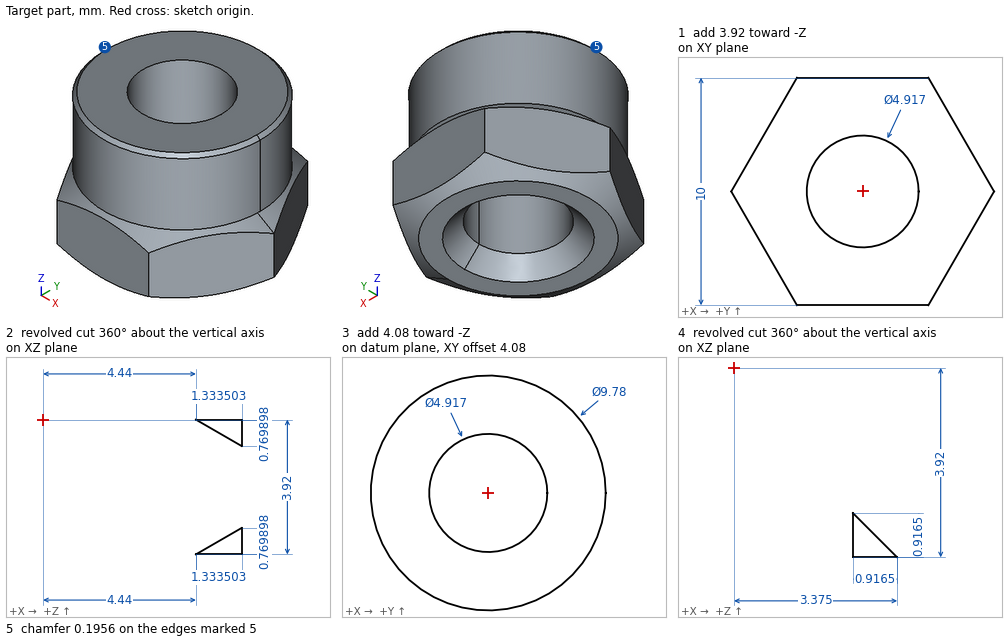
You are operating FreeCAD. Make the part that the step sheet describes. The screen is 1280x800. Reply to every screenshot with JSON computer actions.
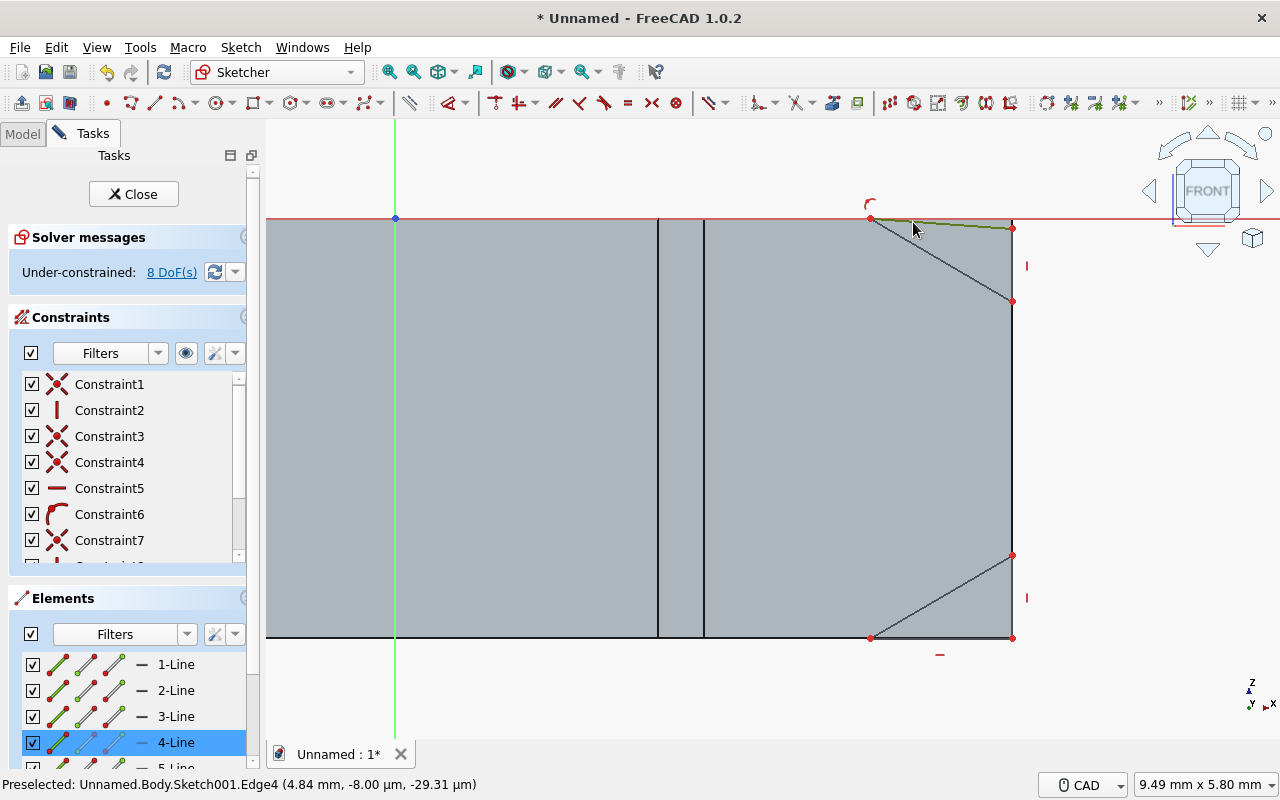
{"action": "key", "text": "h"}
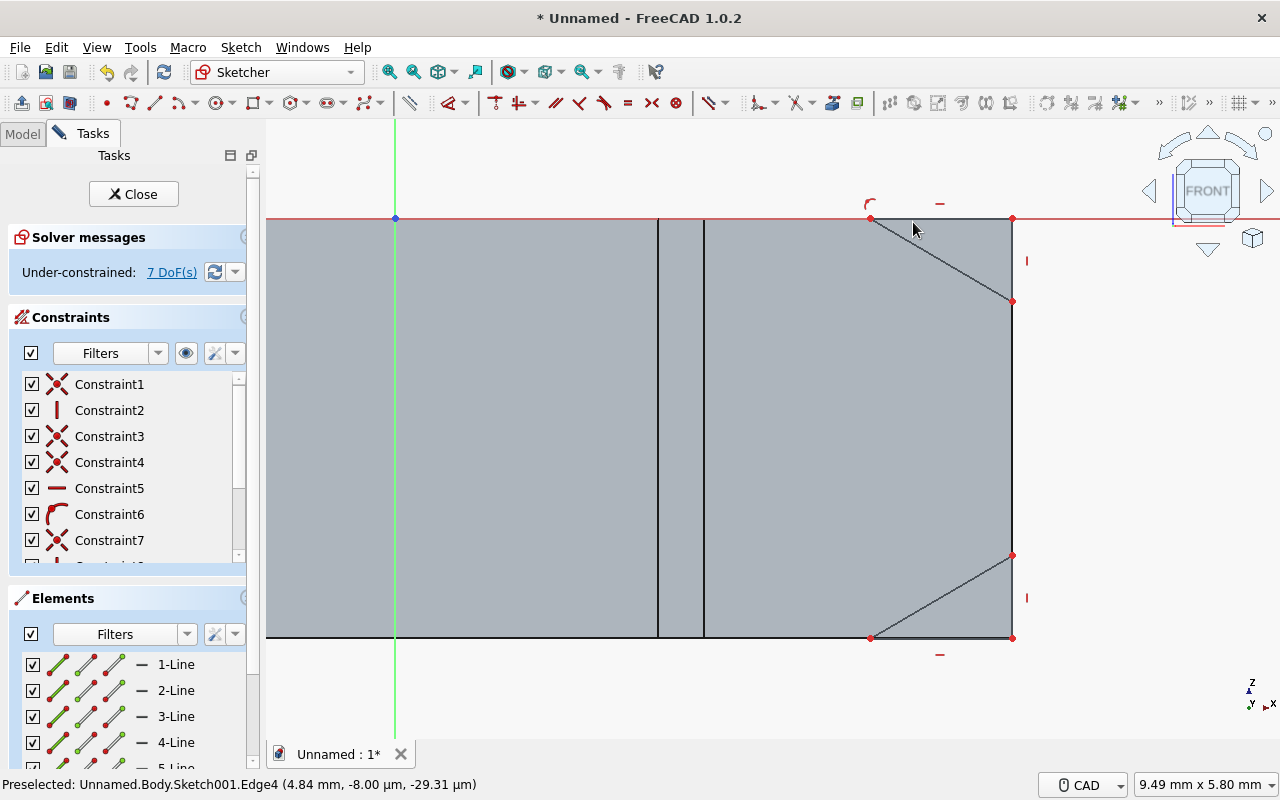
{"action": "key", "text": "d"}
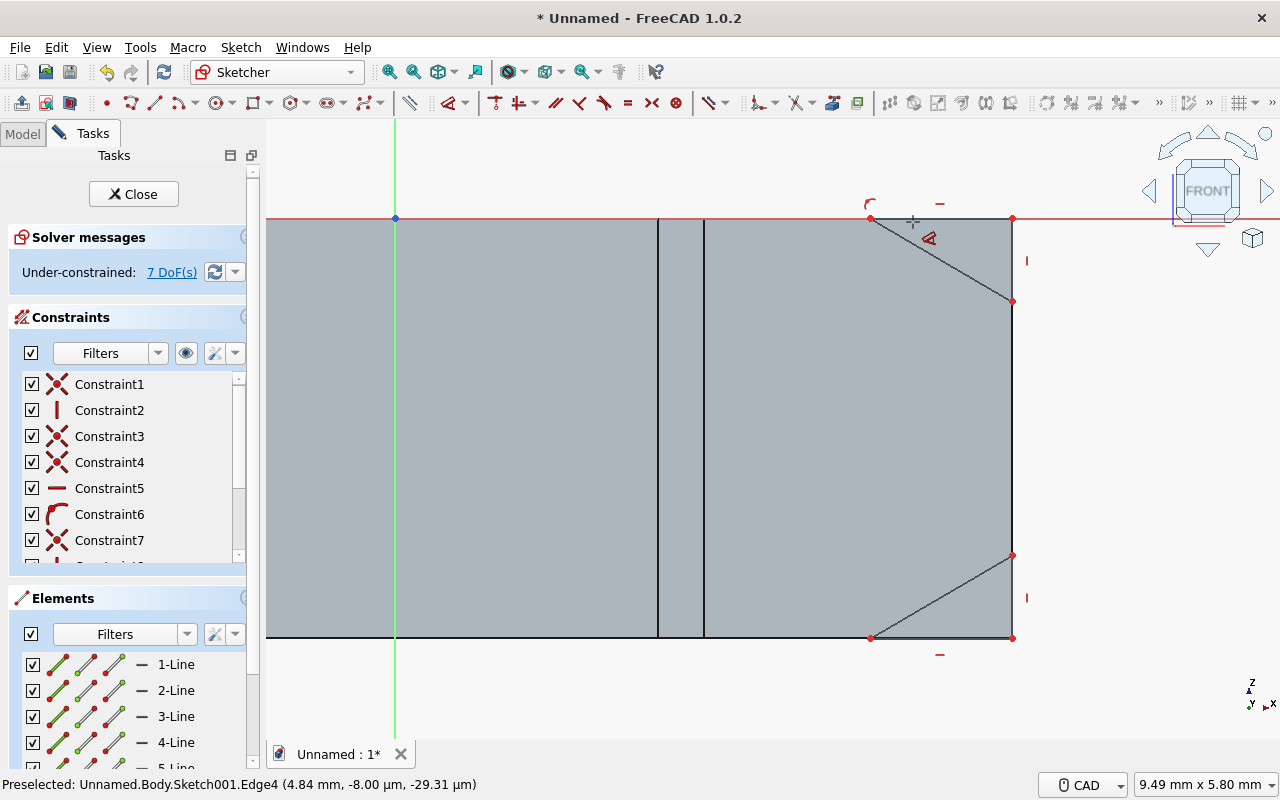
{"action": "left_click", "coordinate": [870, 639]}
{"action": "left_click", "coordinate": [633, 673]}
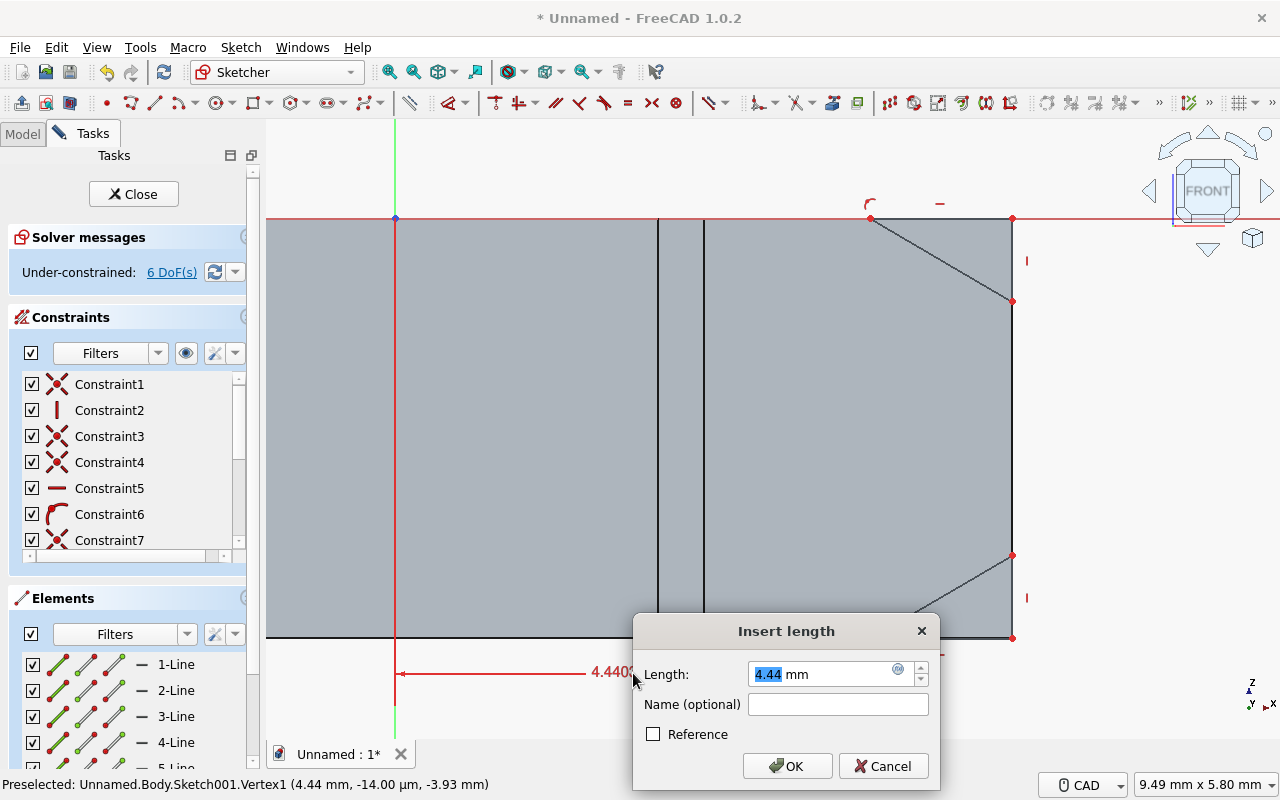
{"action": "type", "text": "4.44"}
{"action": "key", "text": "Return"}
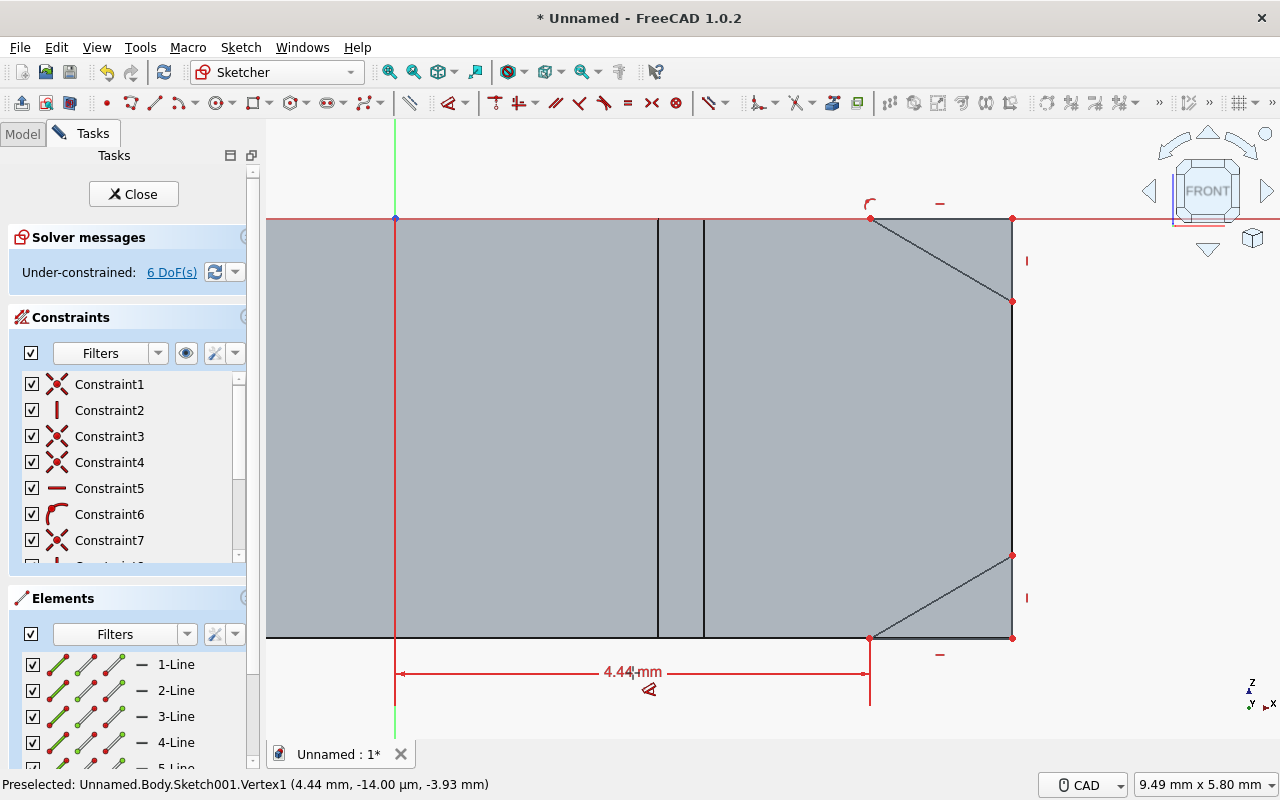
{"action": "left_click", "coordinate": [870, 639]}
{"action": "left_click", "coordinate": [361, 429]}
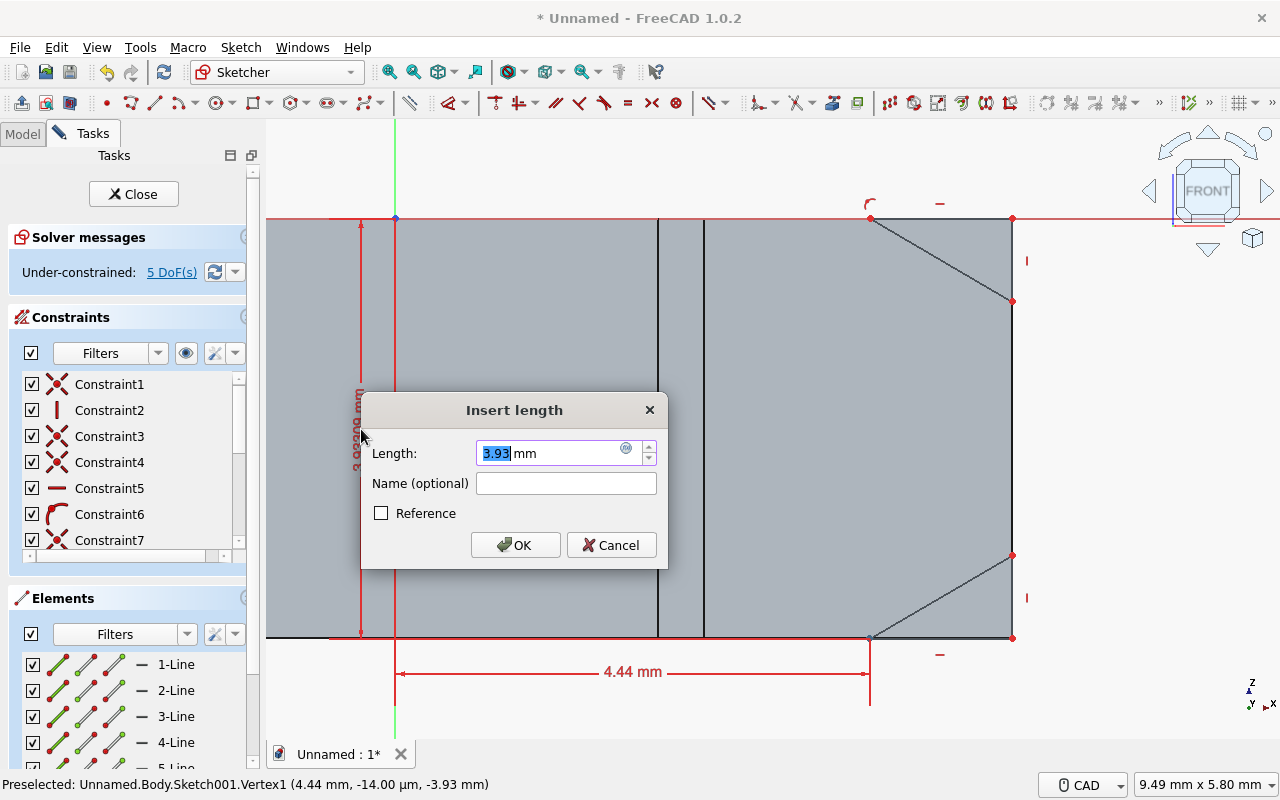
{"action": "type", "text": "3.92"}
{"action": "key", "text": "Return"}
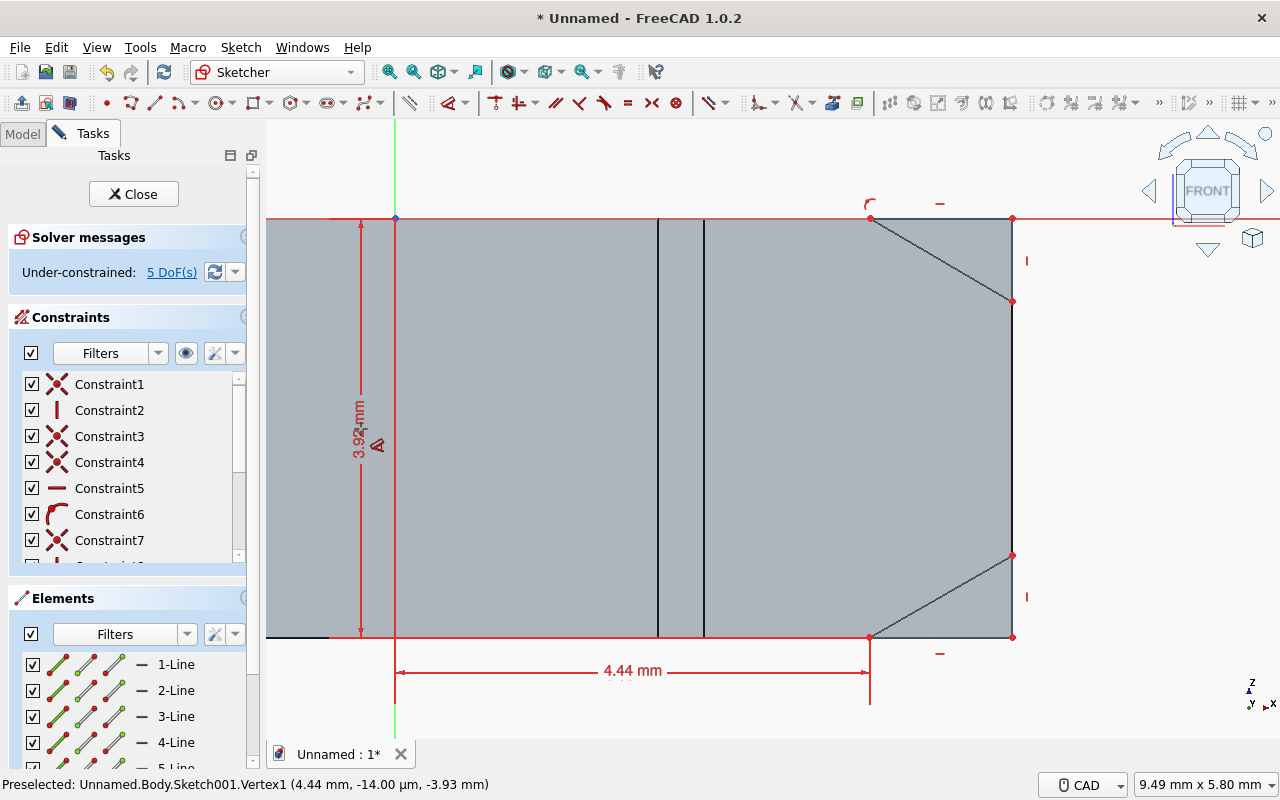
{"action": "left_click", "coordinate": [870, 219]}
{"action": "left_click", "coordinate": [633, 185]}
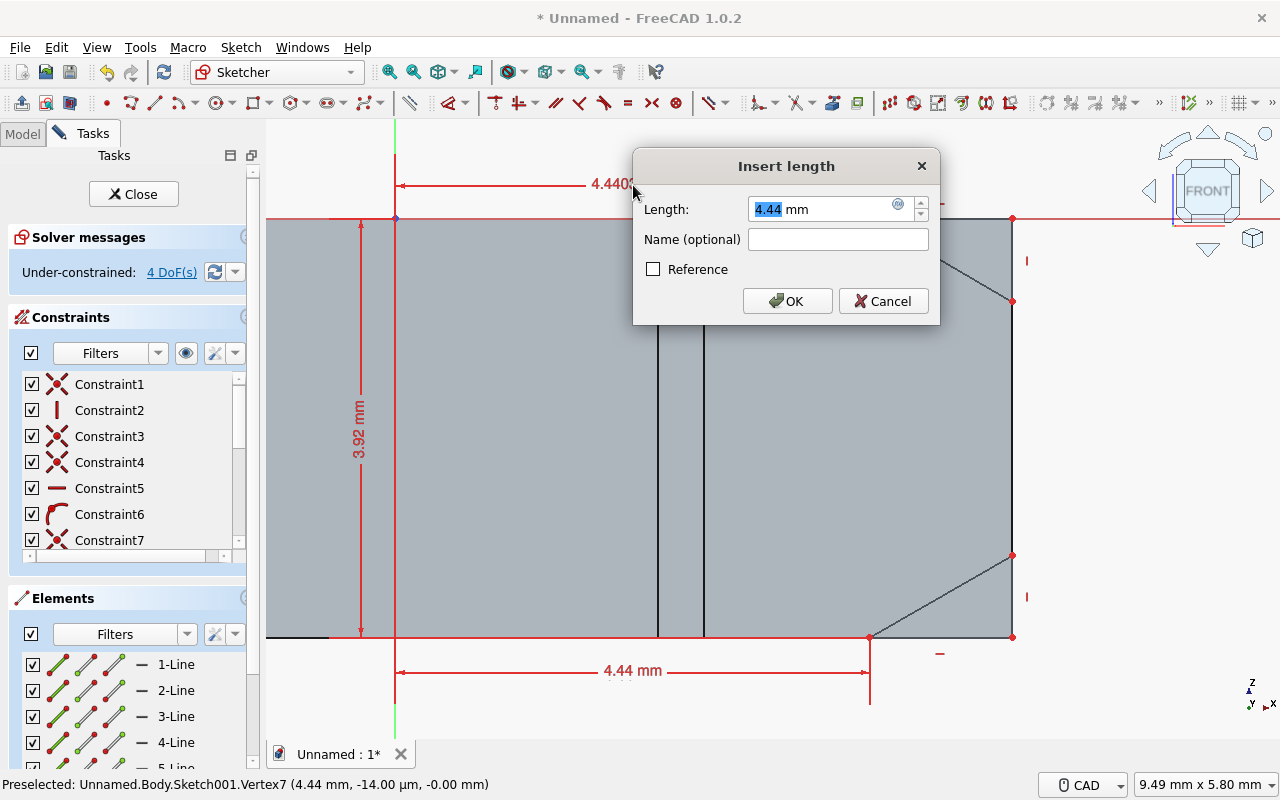
{"action": "type", "text": "4.44"}
{"action": "key", "text": "Return"}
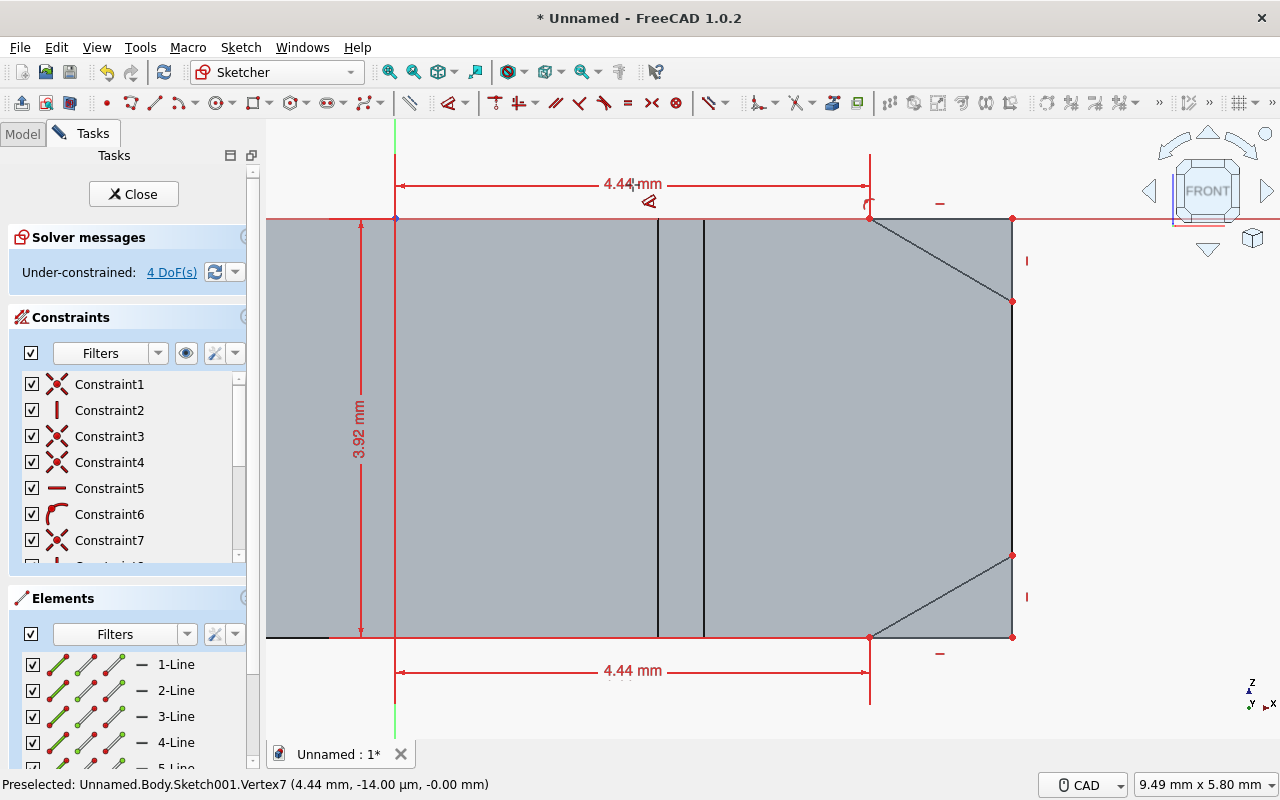
{"action": "left_click", "coordinate": [1012, 580]}
{"action": "left_click", "coordinate": [1046, 597]}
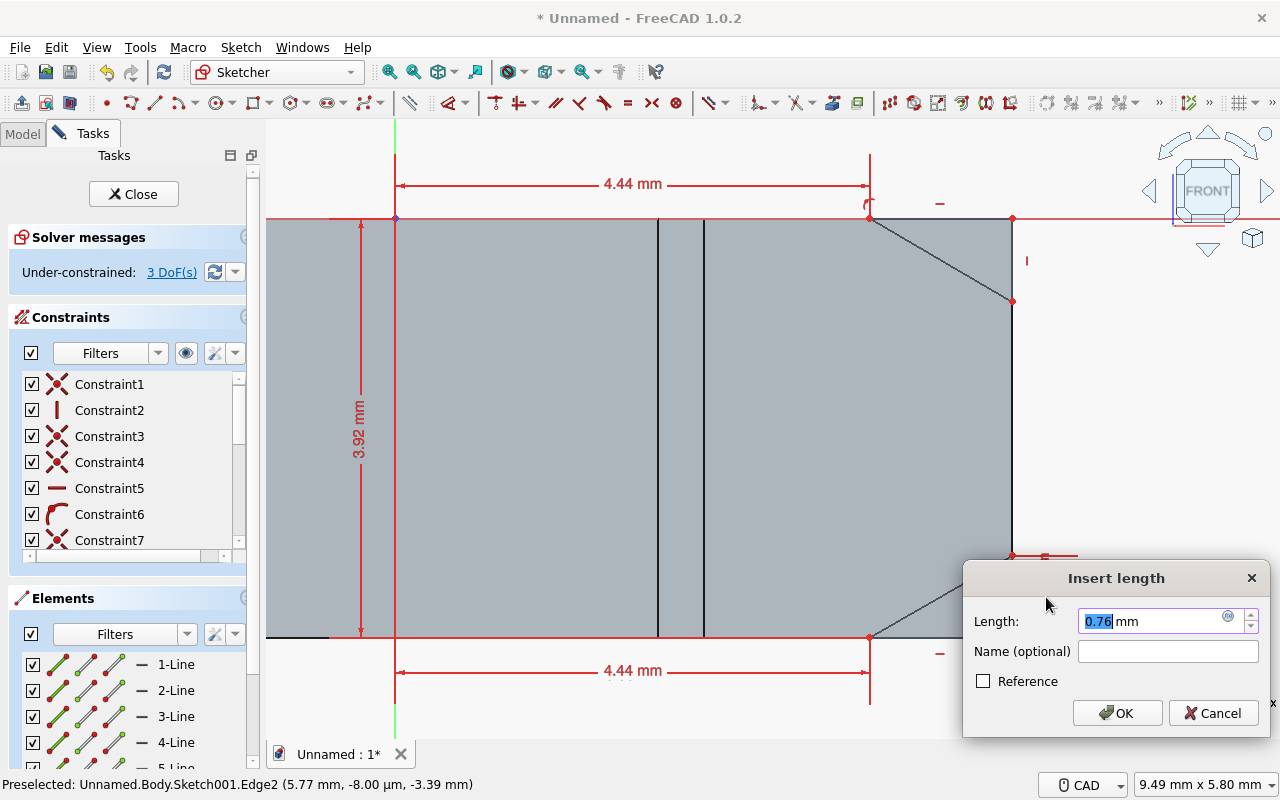
{"action": "type", "text": "0.769898"}
{"action": "key", "text": "Return"}